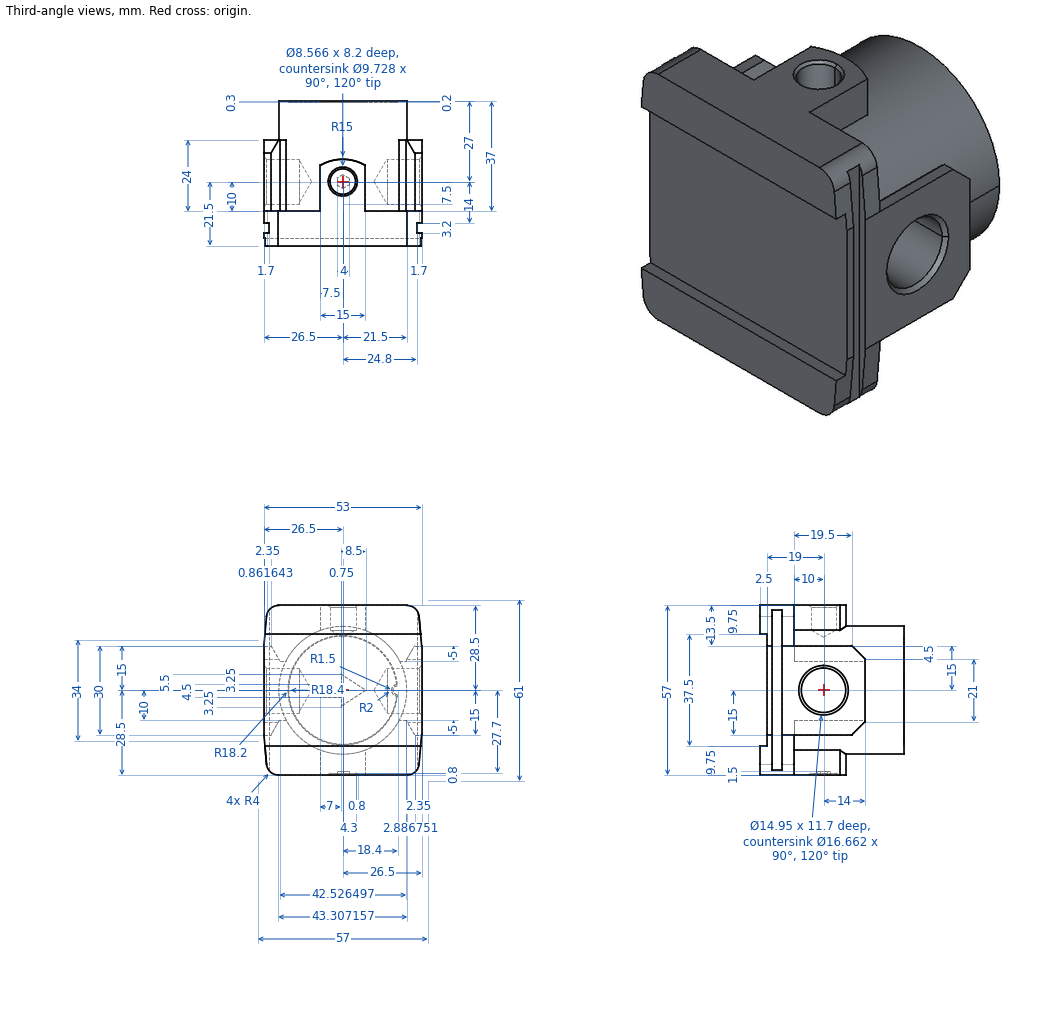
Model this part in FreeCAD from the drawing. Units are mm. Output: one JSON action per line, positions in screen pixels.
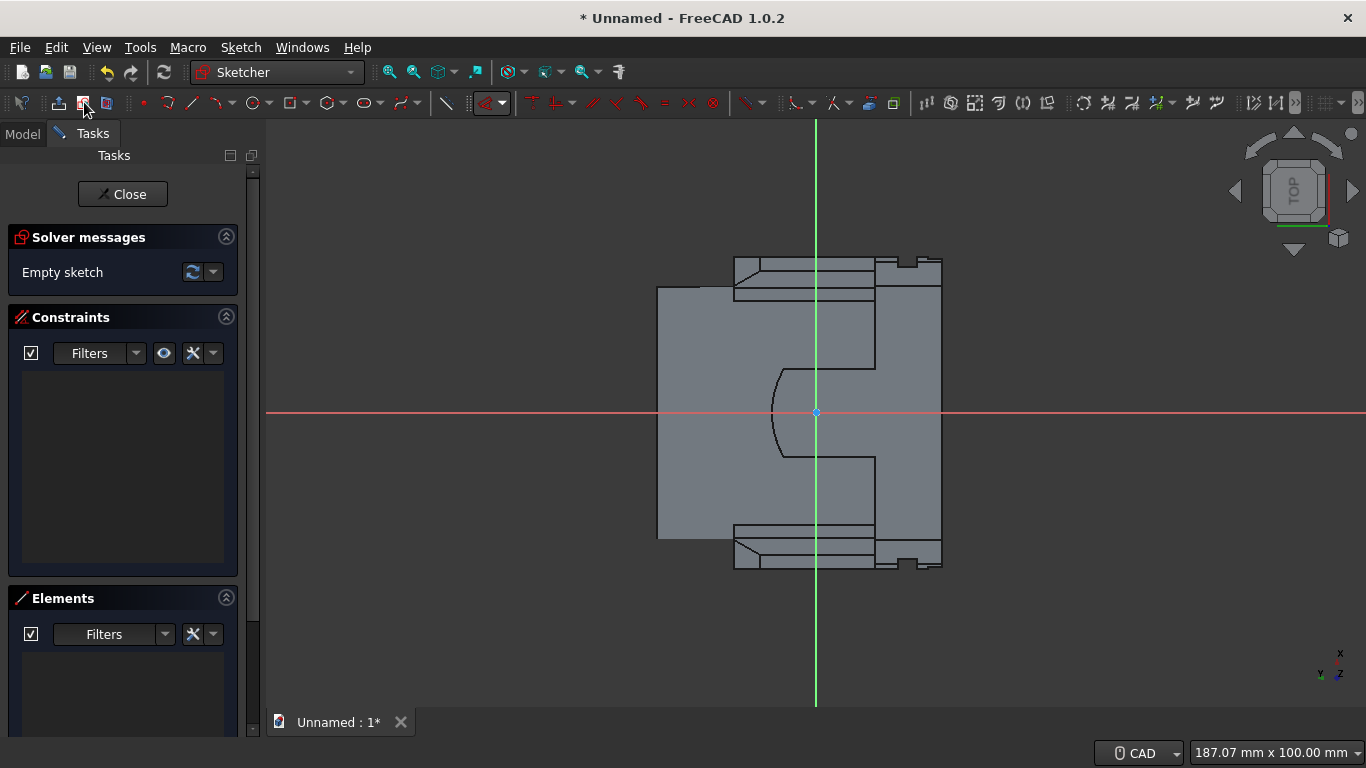
{"action": "scroll", "coordinate": [827, 413], "scroll_direction": "up", "scroll_amount": 10}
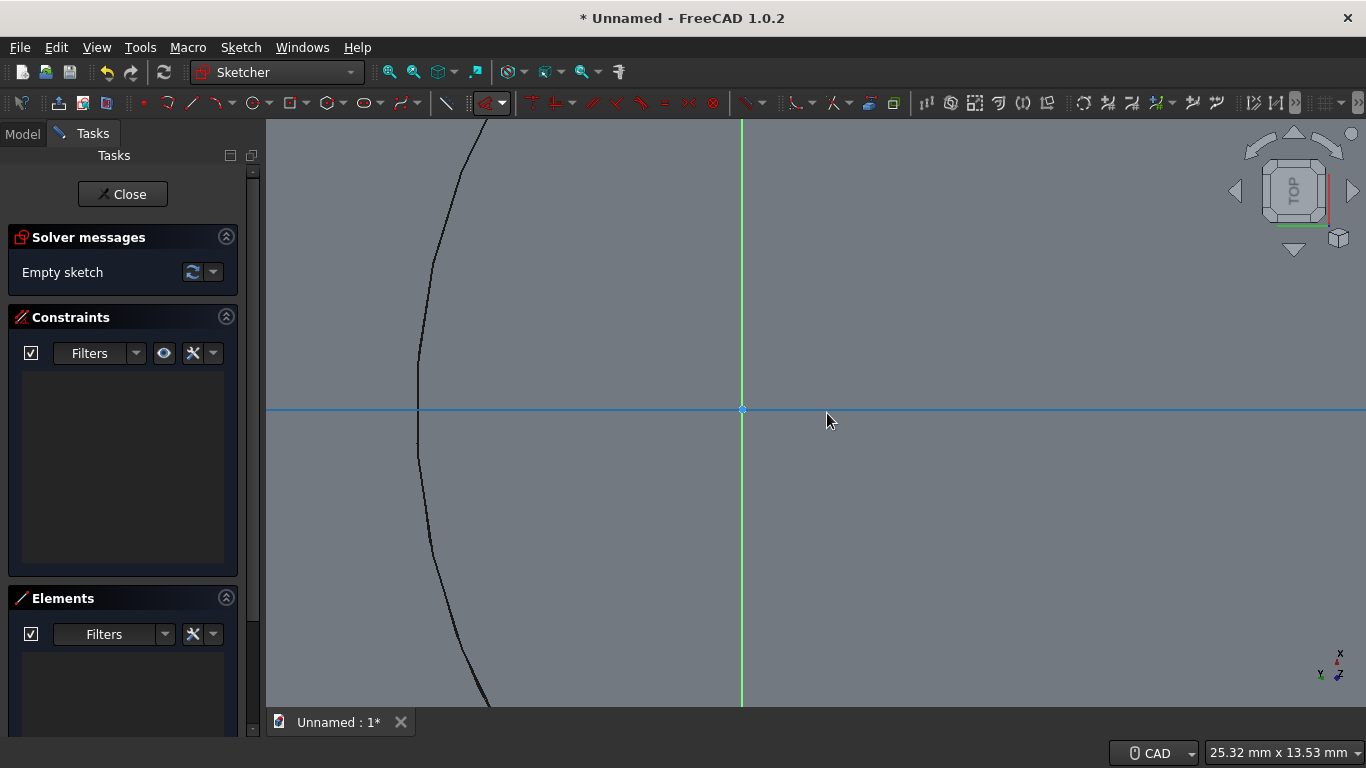
{"action": "left_click", "coordinate": [254, 104]}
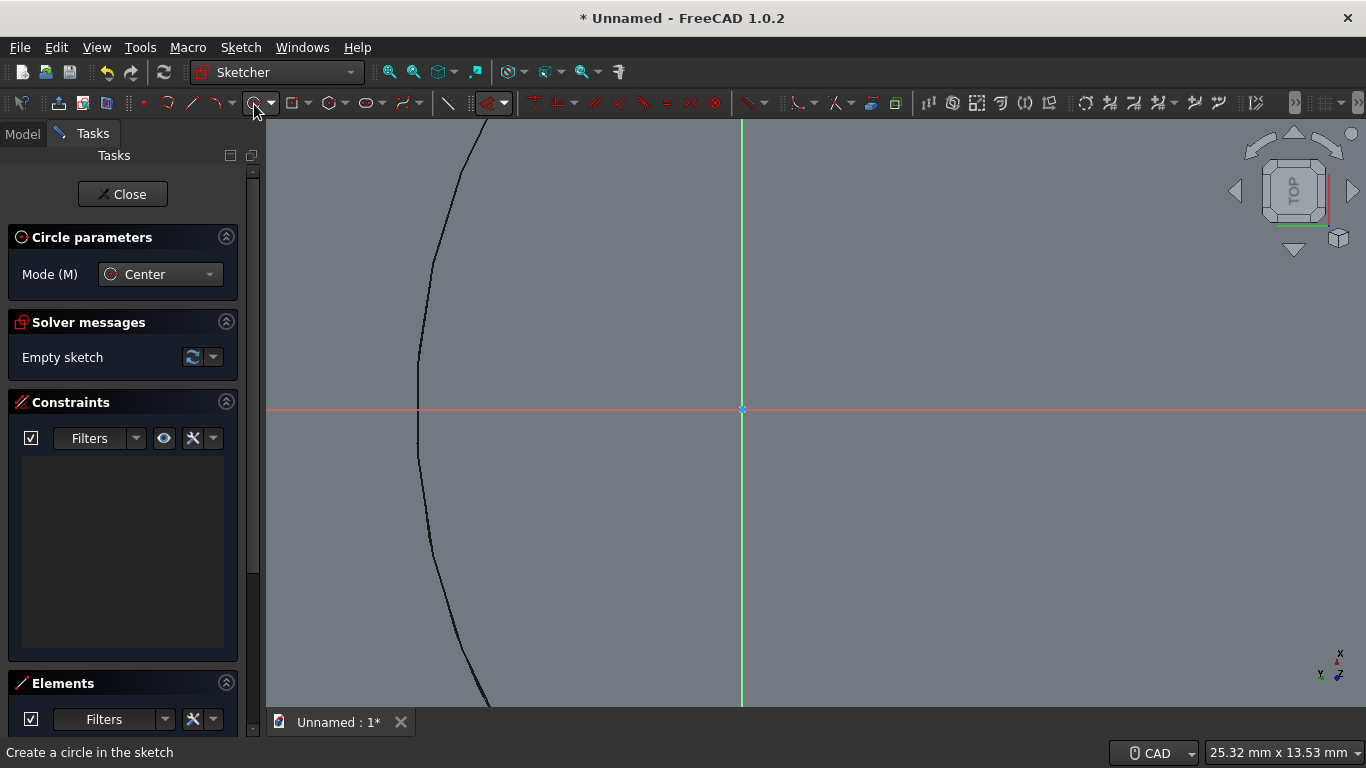
{"action": "left_click", "coordinate": [742, 410]}
{"action": "mouse_move", "coordinate": [874, 278]}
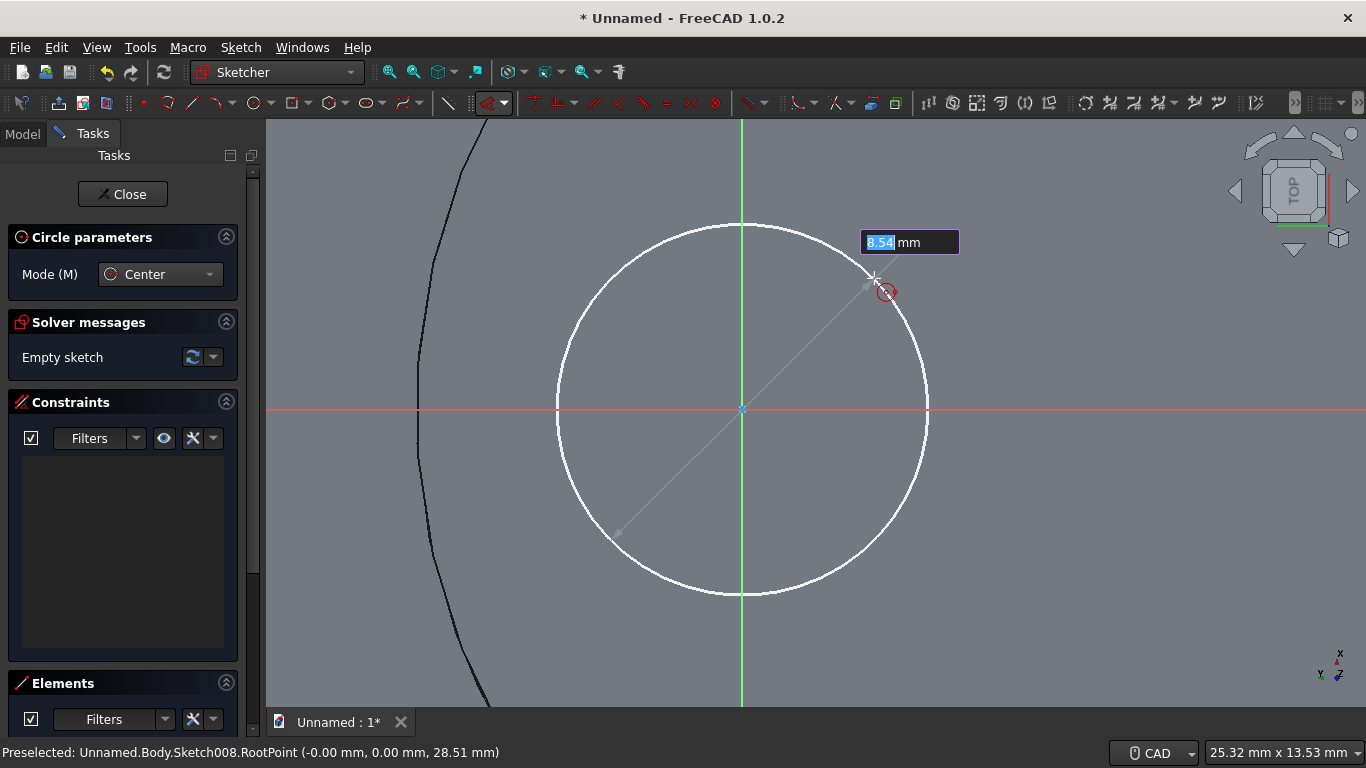
{"action": "type", "text": "8.566"}
{"action": "key", "text": "Return"}
{"action": "key", "text": "Escape"}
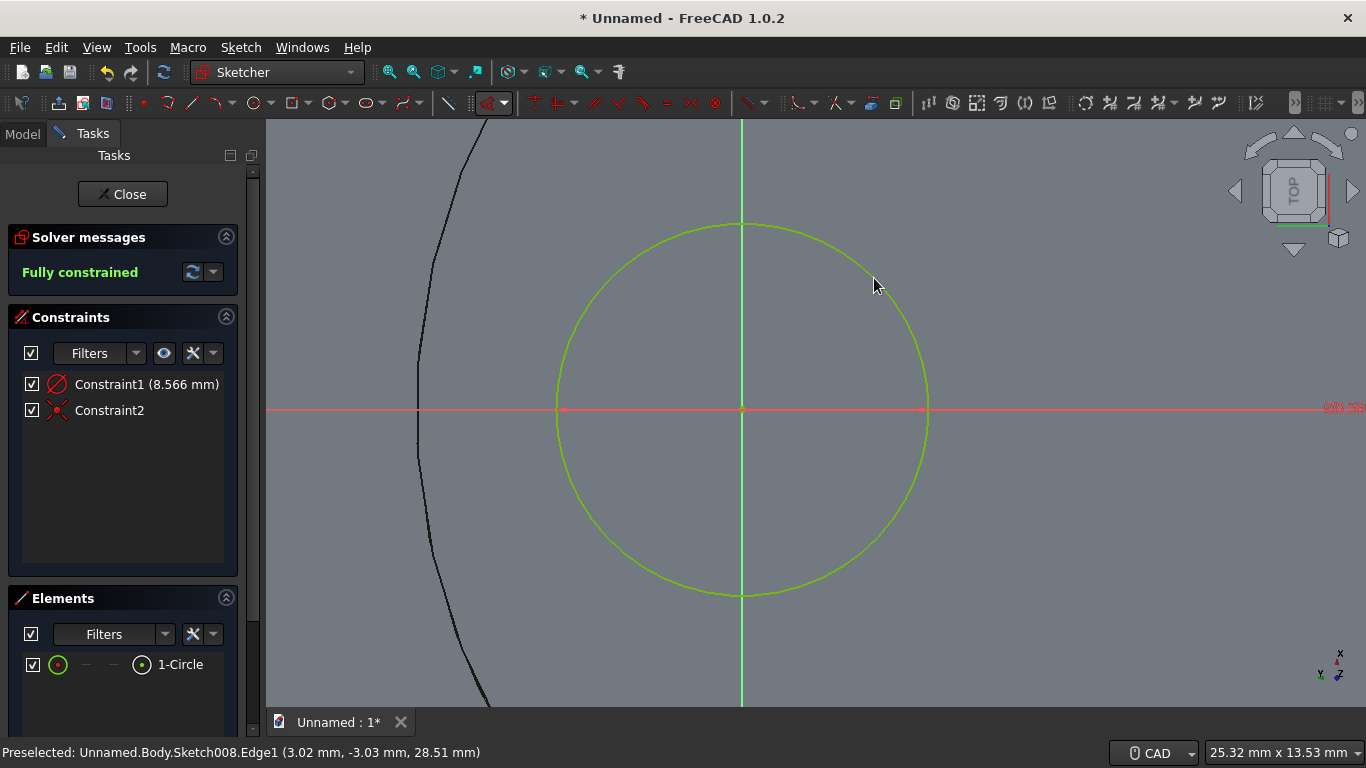
{"action": "left_click", "coordinate": [123, 194]}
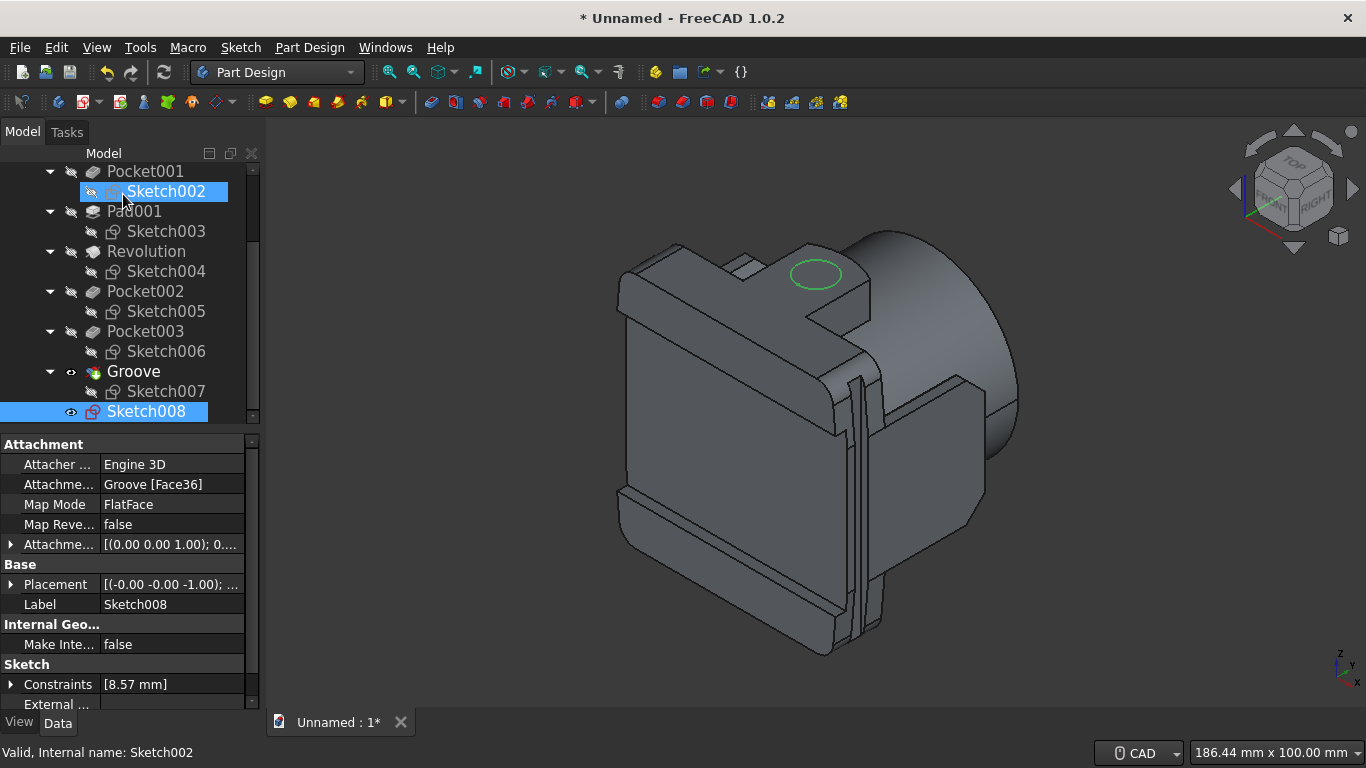
{"action": "left_click", "coordinate": [456, 102]}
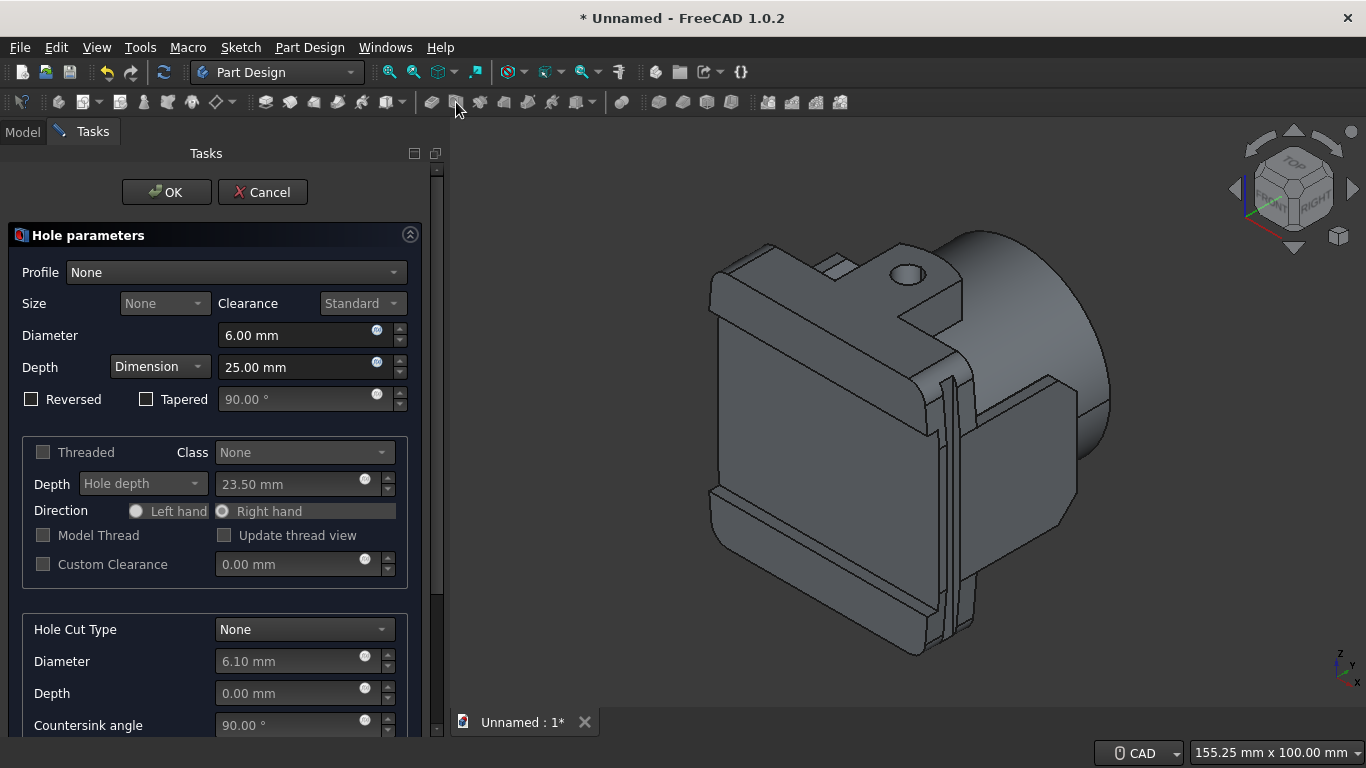
{"action": "triple_click", "coordinate": [305, 335]}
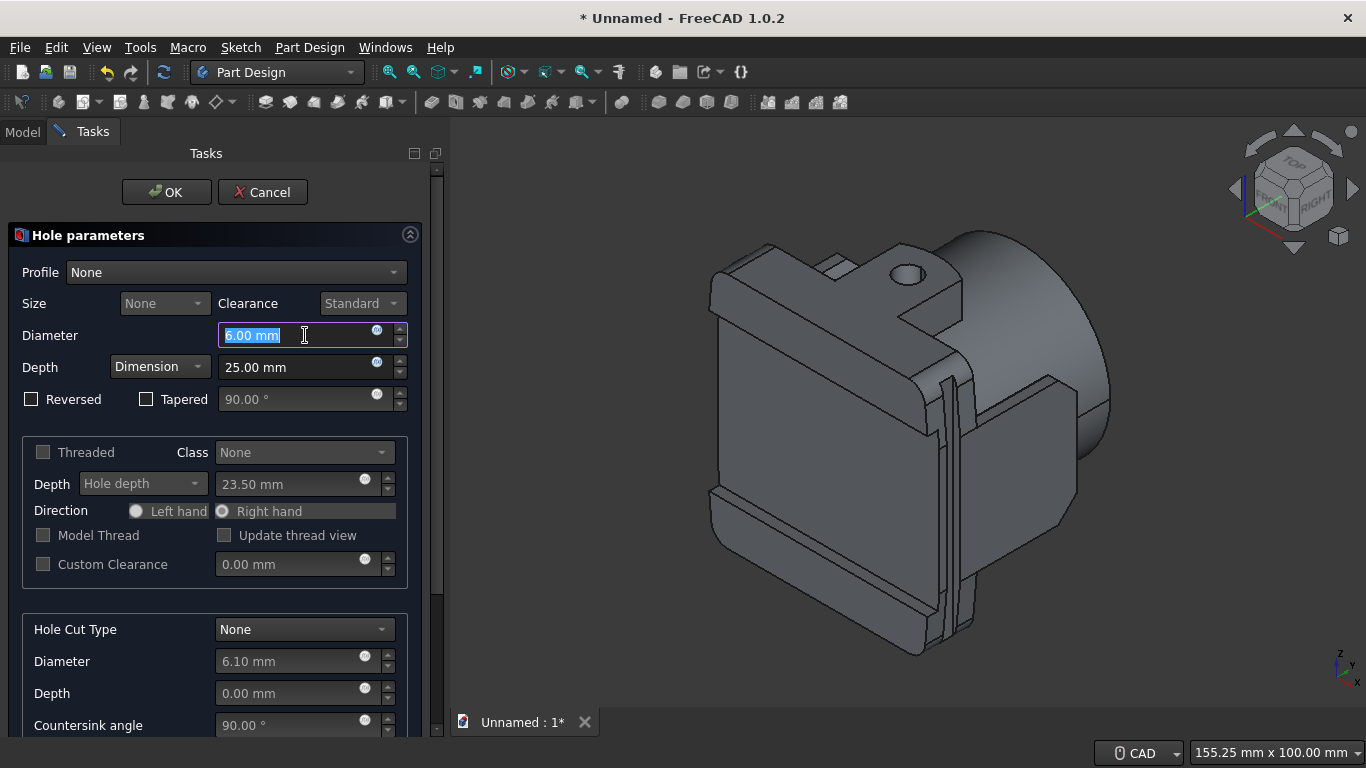
{"action": "type", "text": "8.566"}
{"action": "key", "text": "Tab"}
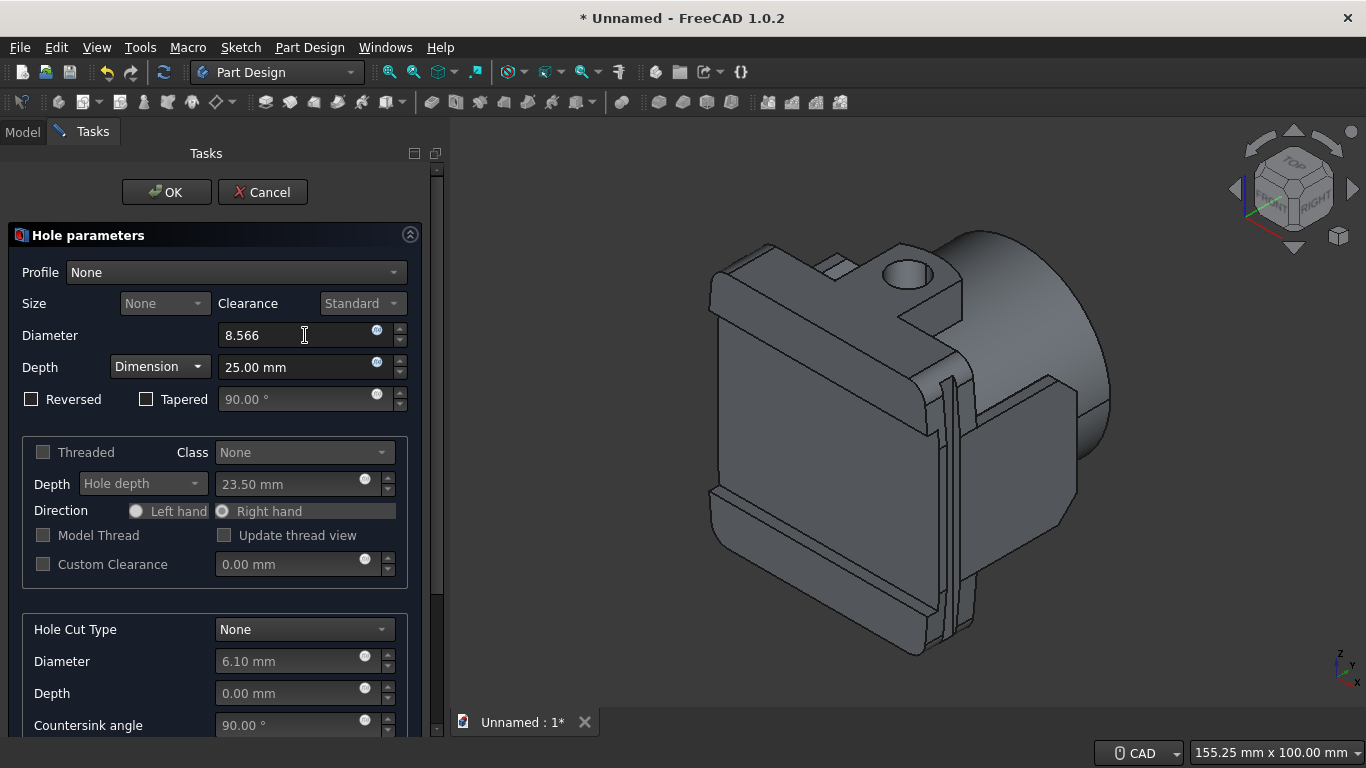
{"action": "triple_click", "coordinate": [305, 367]}